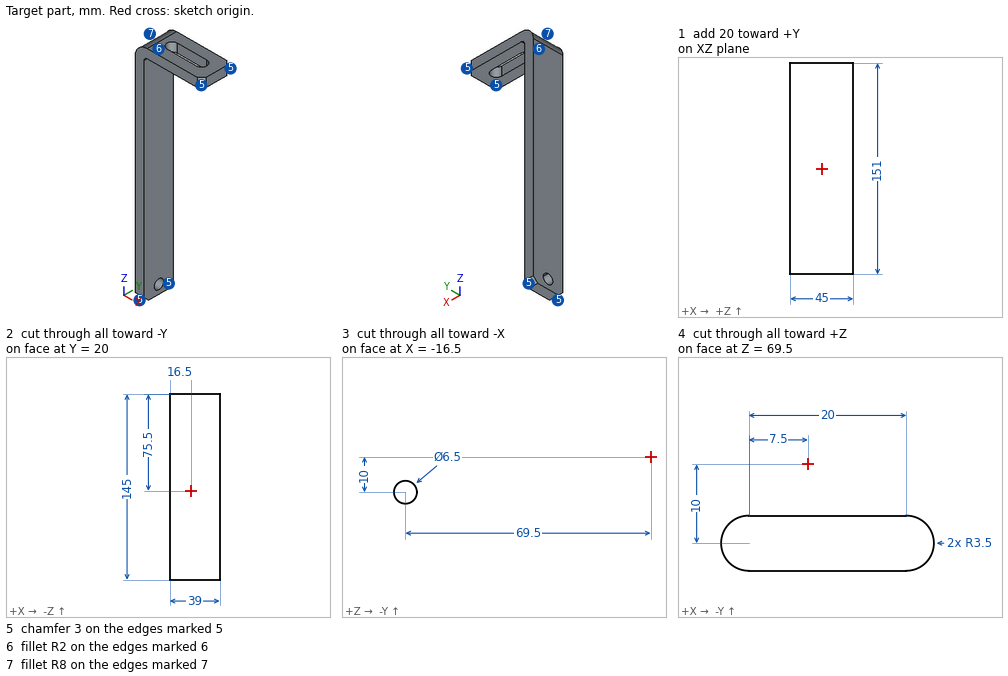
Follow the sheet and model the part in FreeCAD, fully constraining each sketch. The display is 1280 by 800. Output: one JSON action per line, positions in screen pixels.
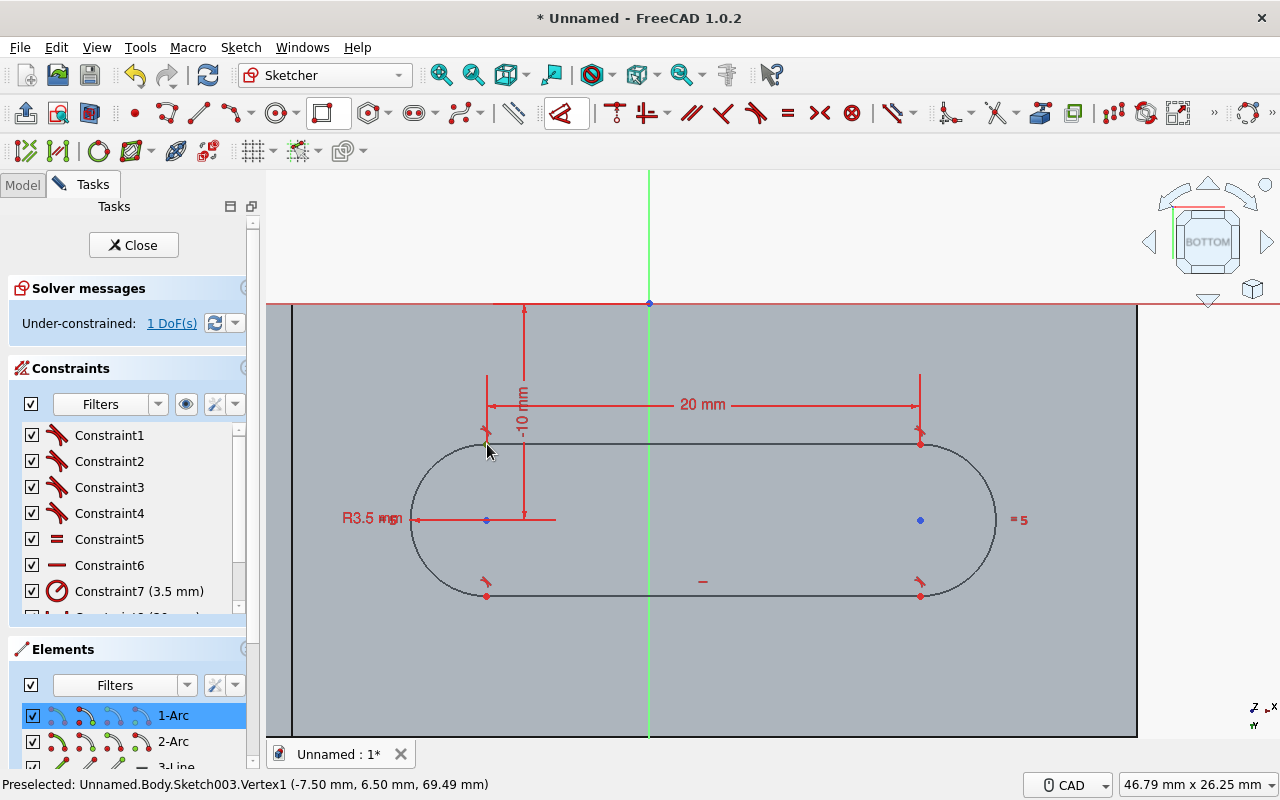
{"action": "left_click", "coordinate": [584, 114]}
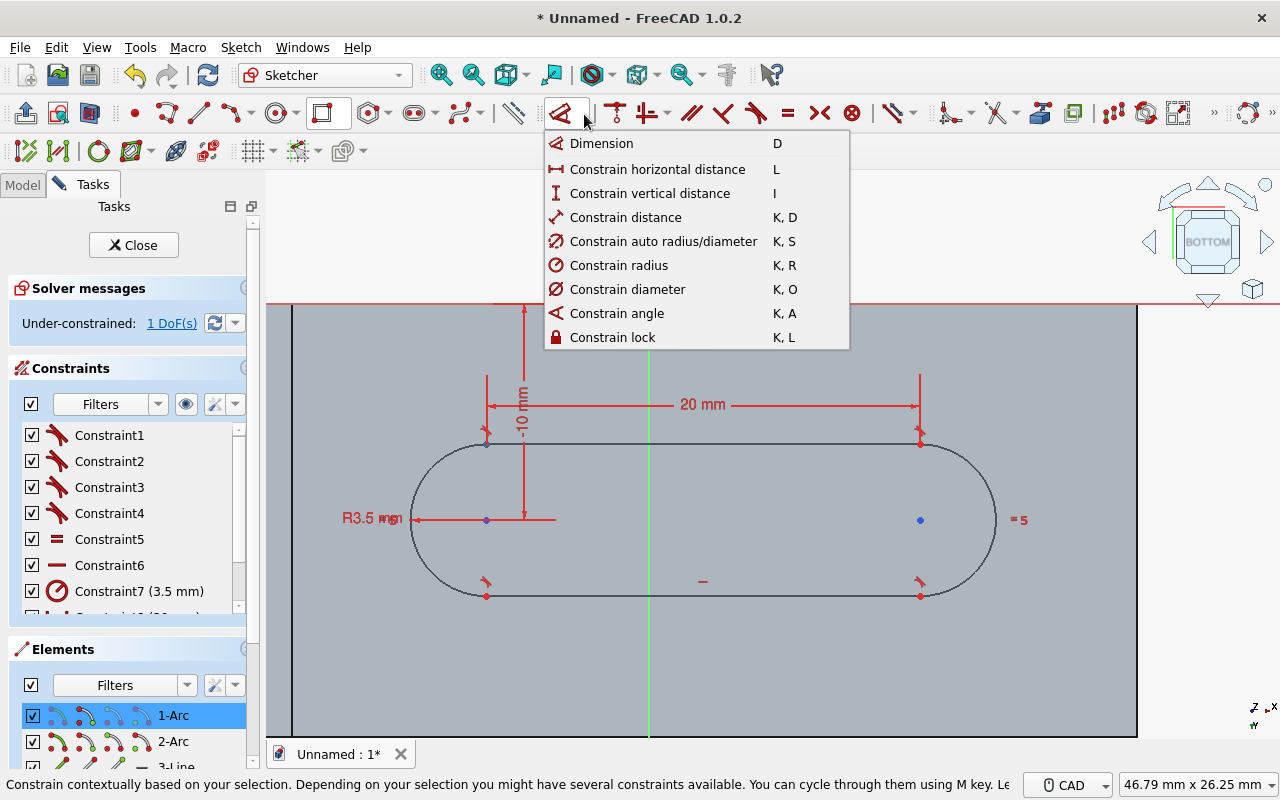
{"action": "left_click", "coordinate": [697, 169]}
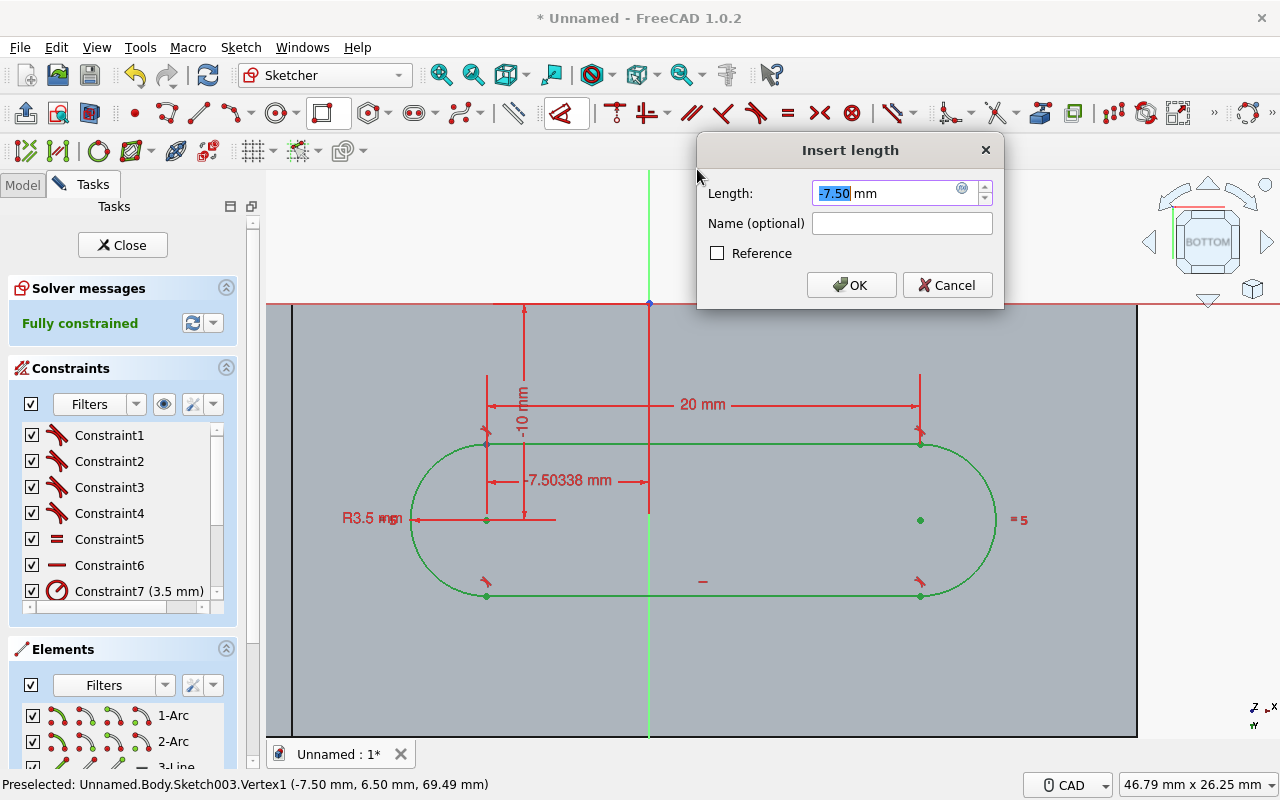
{"action": "type", "text": "-7.5"}
{"action": "key", "text": "Return"}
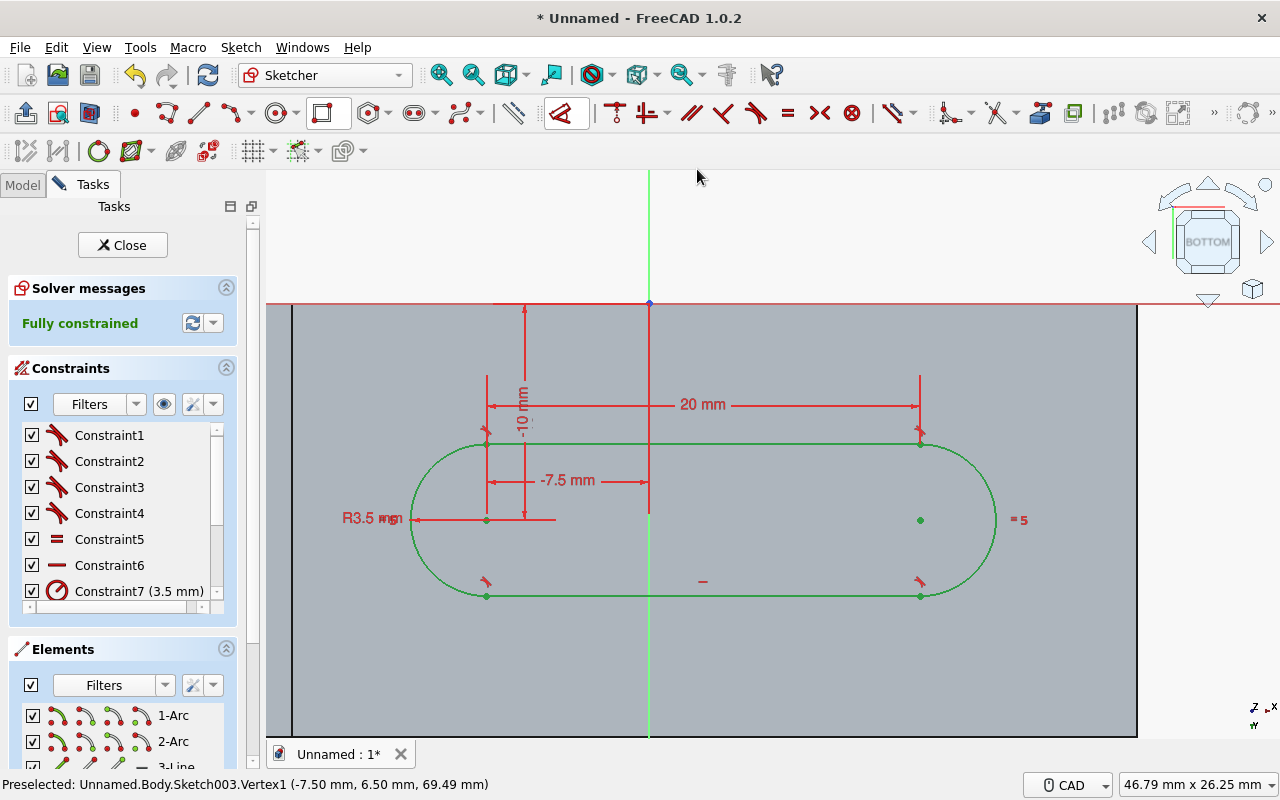
{"action": "left_click", "coordinate": [123, 245]}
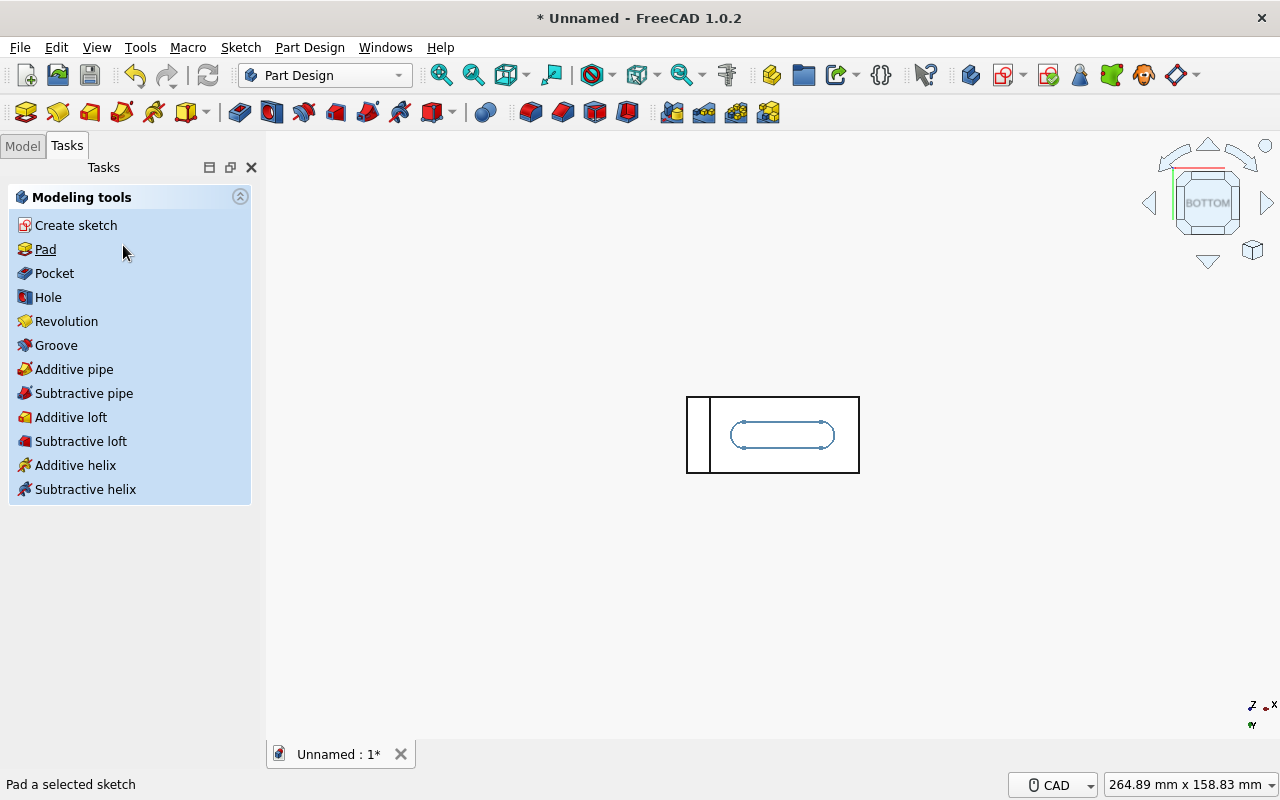
{"action": "left_click", "coordinate": [240, 112]}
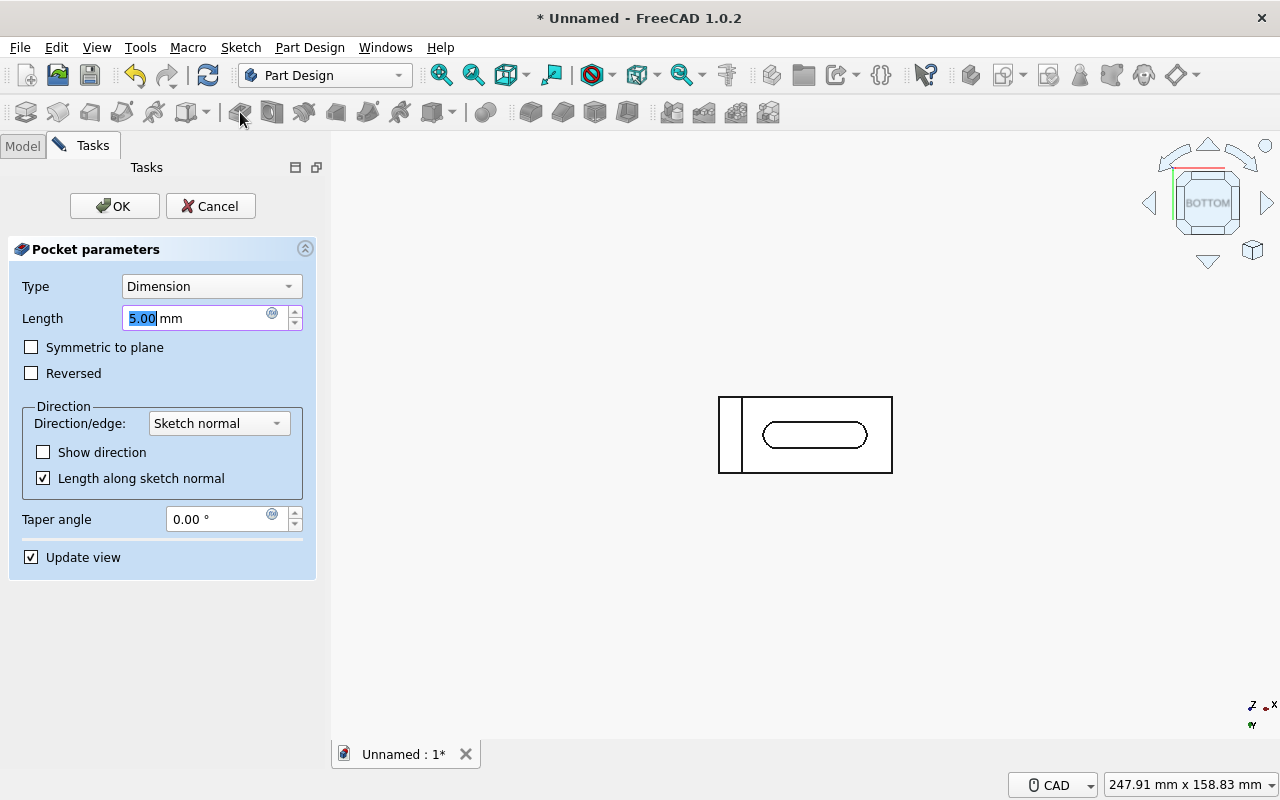
{"action": "left_click", "coordinate": [212, 286]}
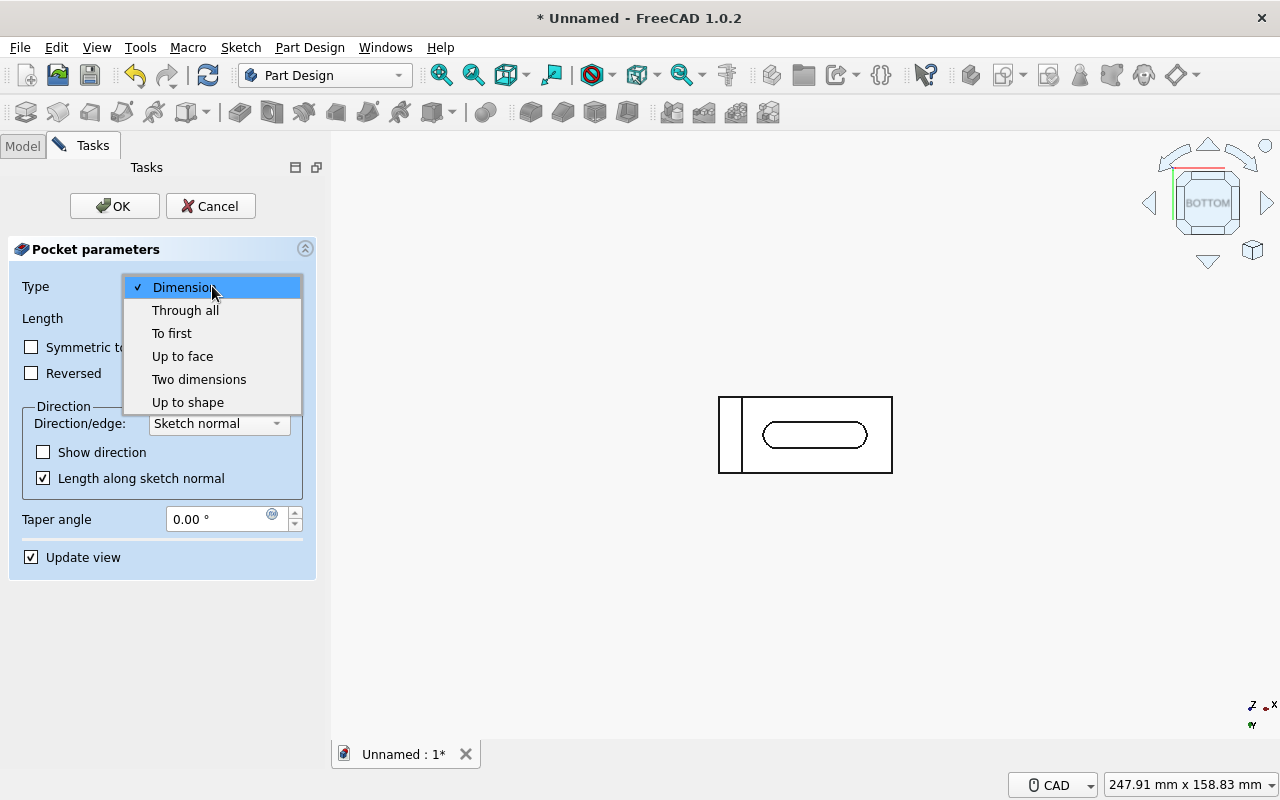
{"action": "left_click", "coordinate": [212, 310]}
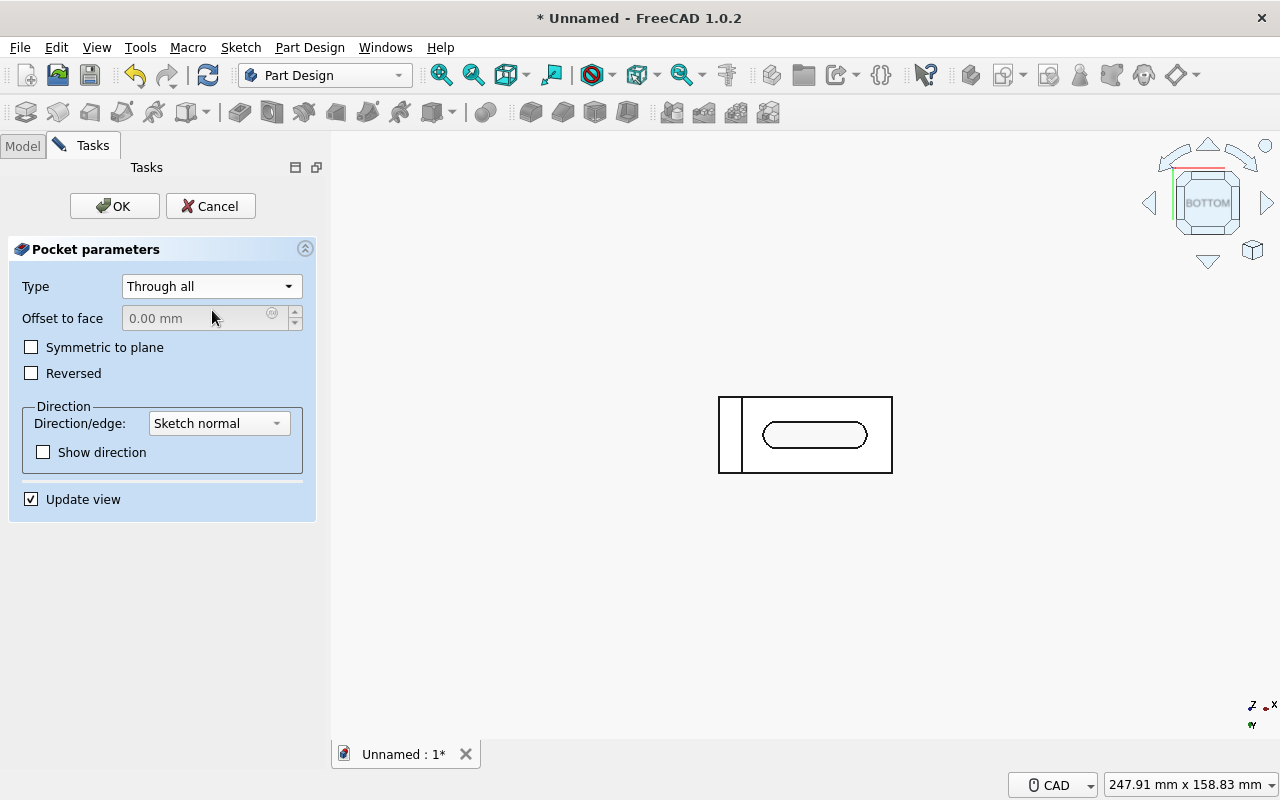
{"action": "left_click", "coordinate": [115, 206]}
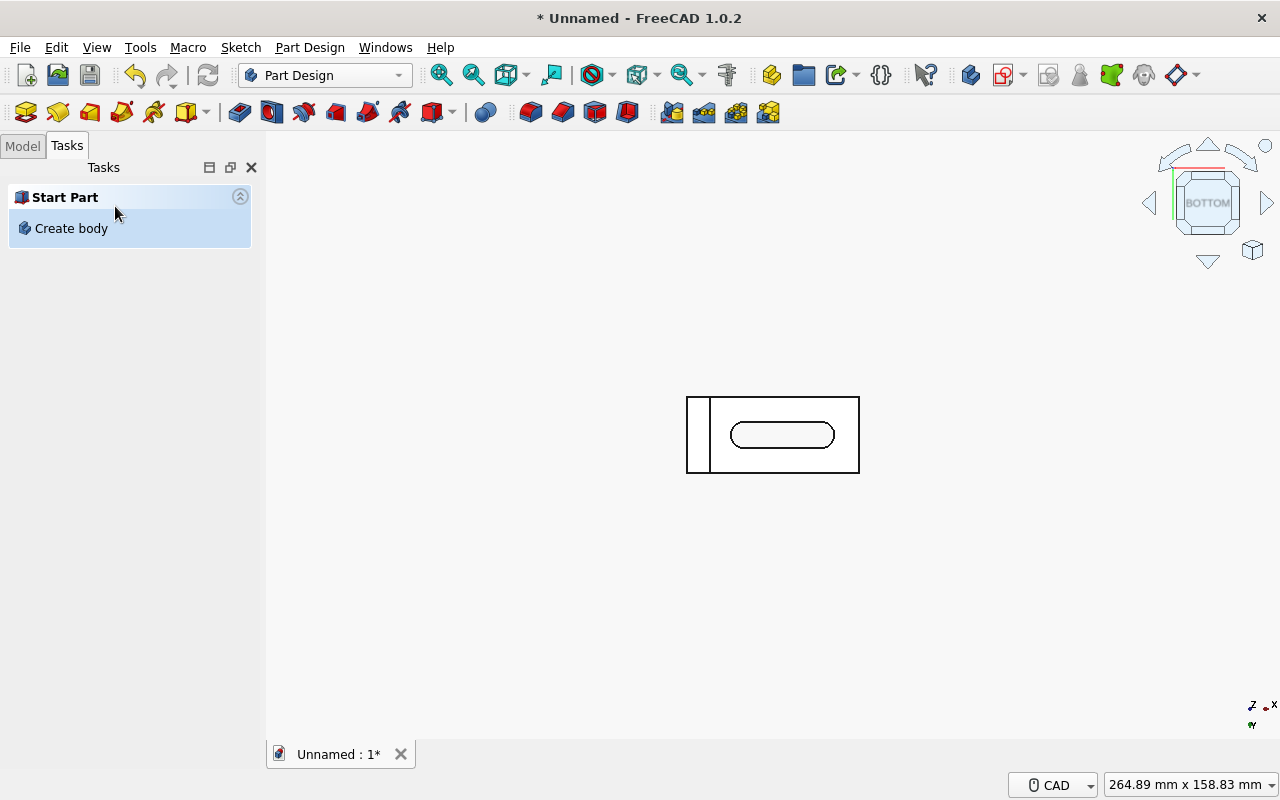
{"action": "left_click", "coordinate": [442, 76]}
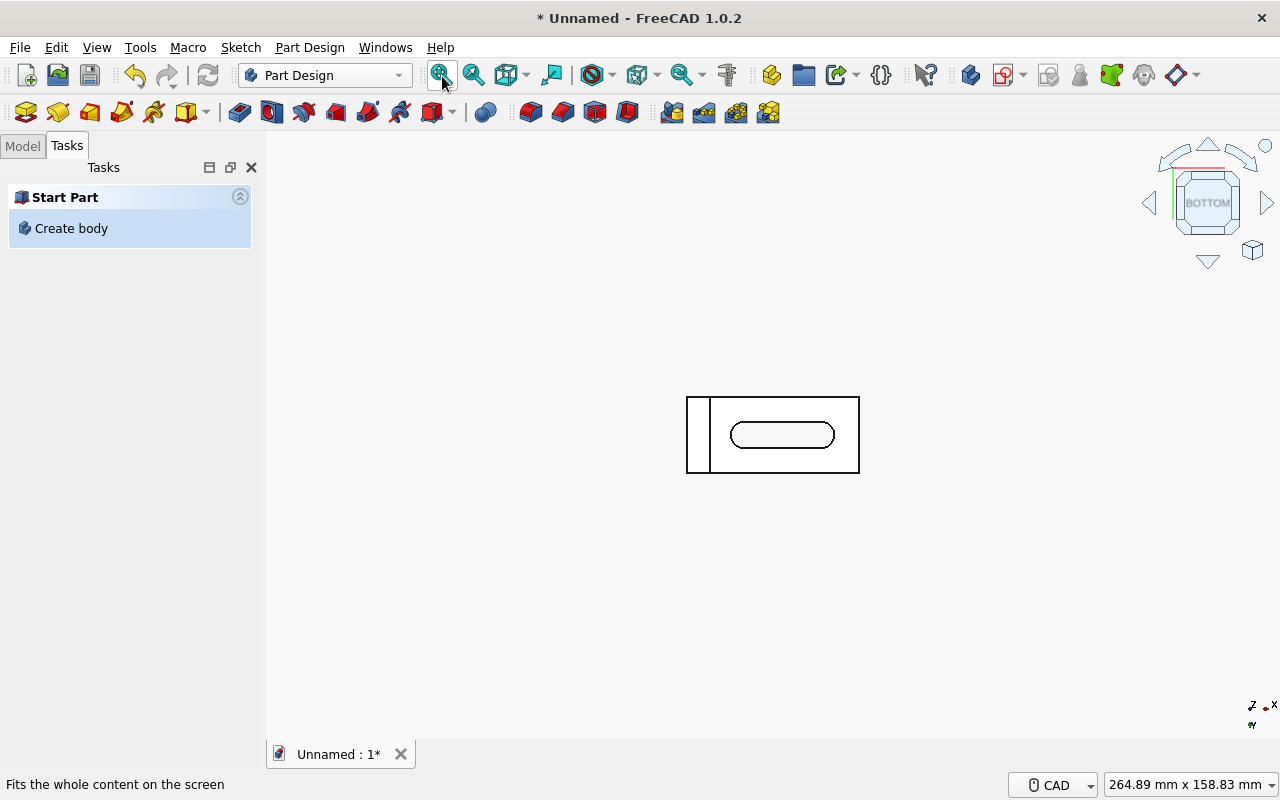
{"action": "left_click", "coordinate": [698, 396]}